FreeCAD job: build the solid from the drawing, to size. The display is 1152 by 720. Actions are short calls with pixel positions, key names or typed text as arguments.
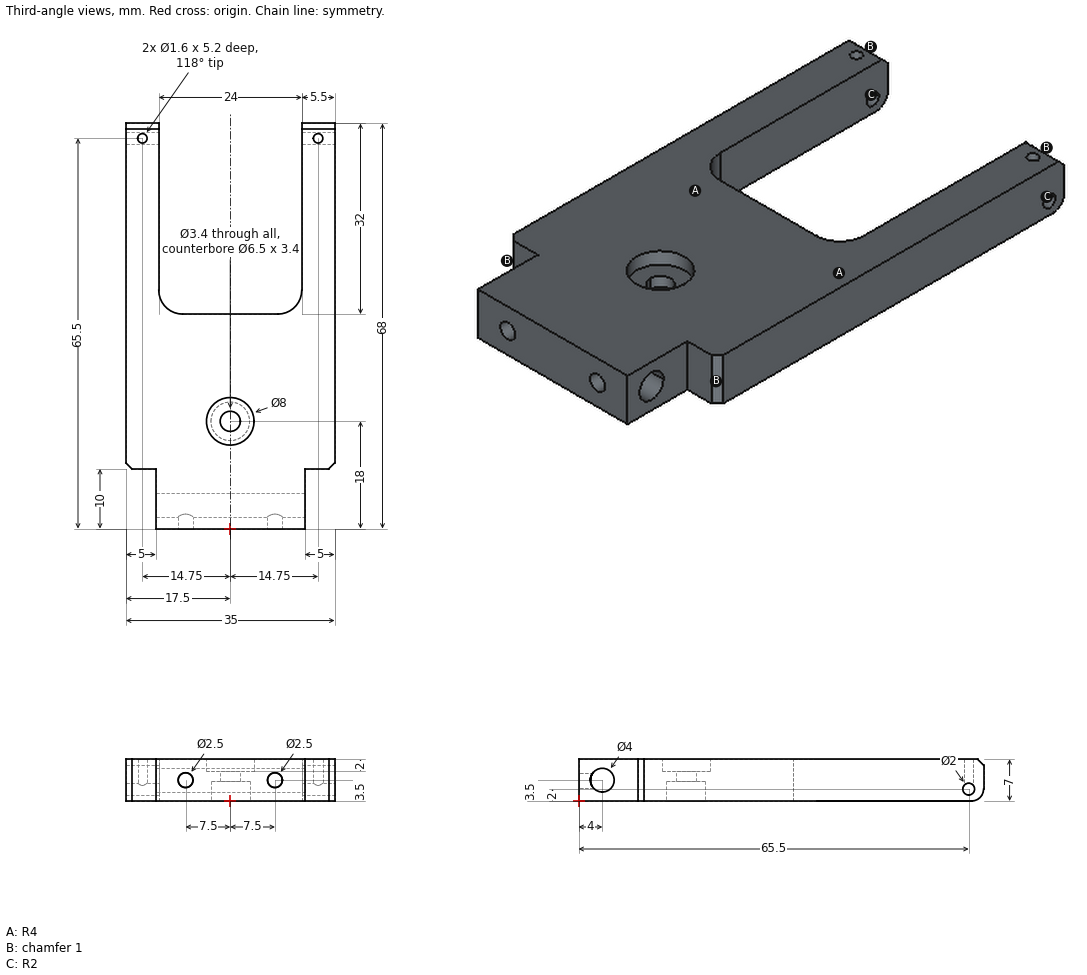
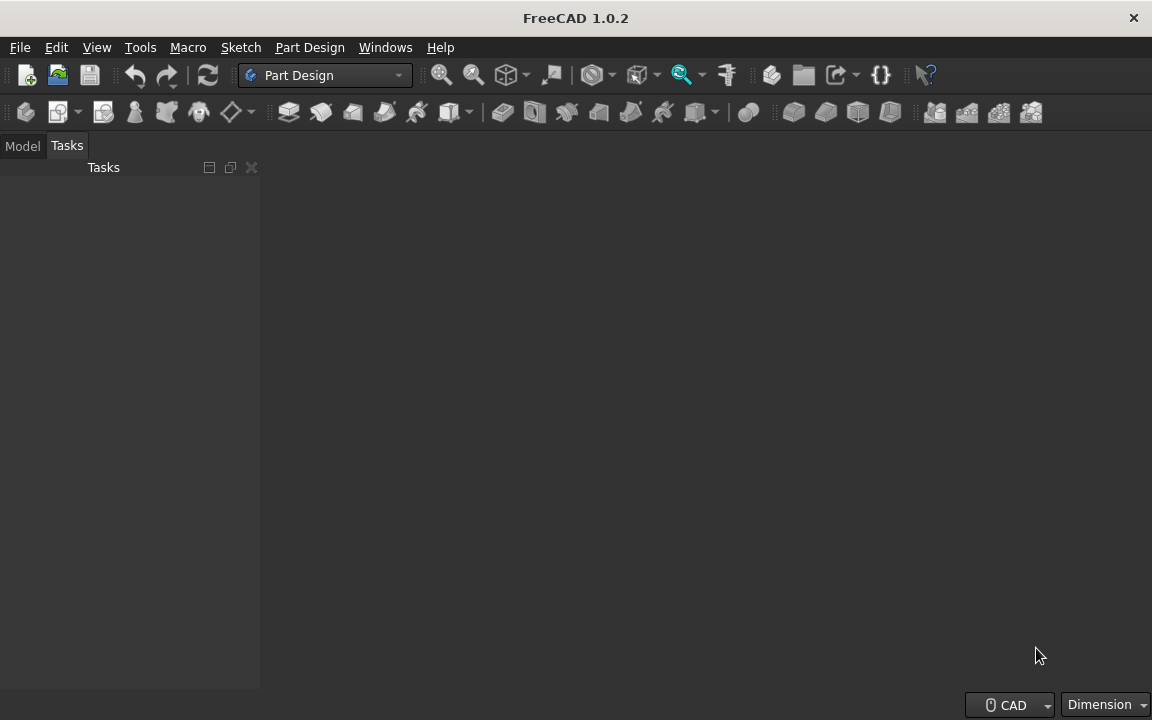
key(ctrl+n)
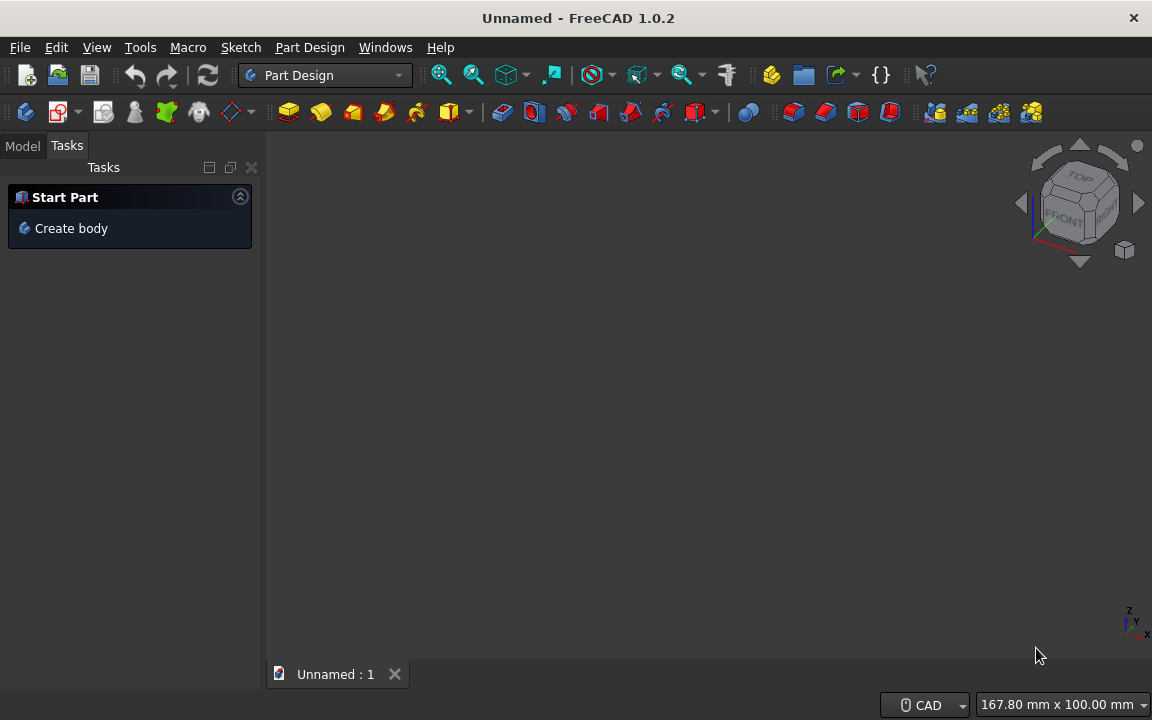
click(58, 112)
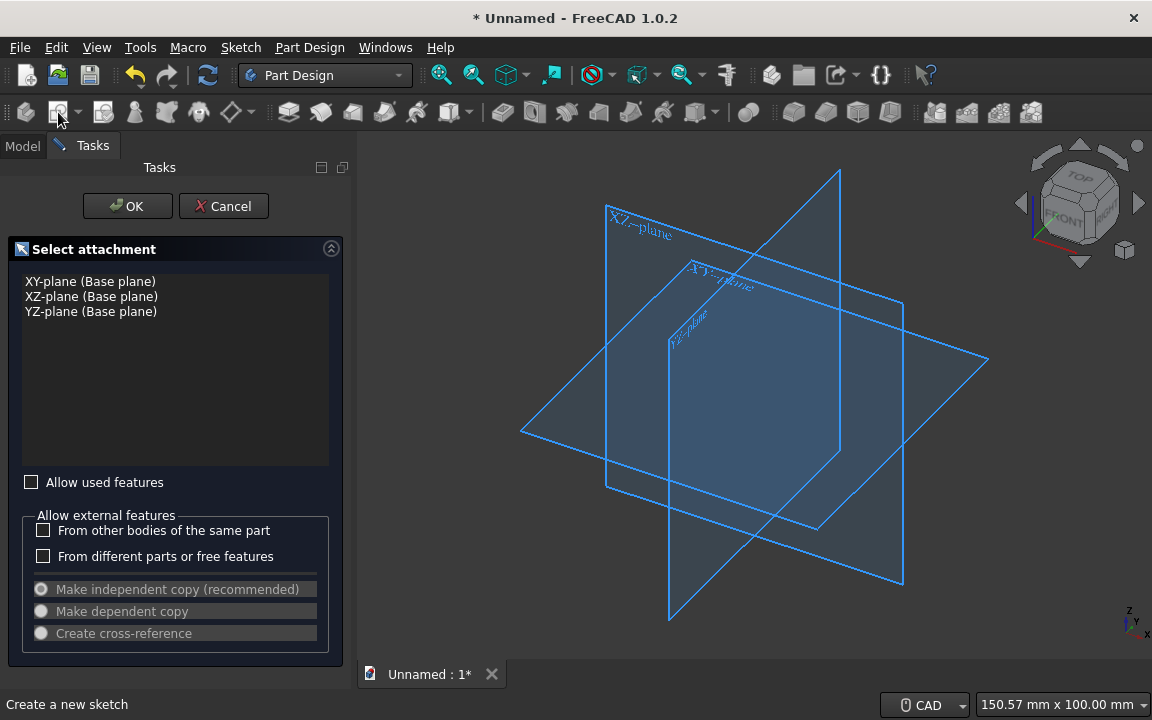
click(82, 282)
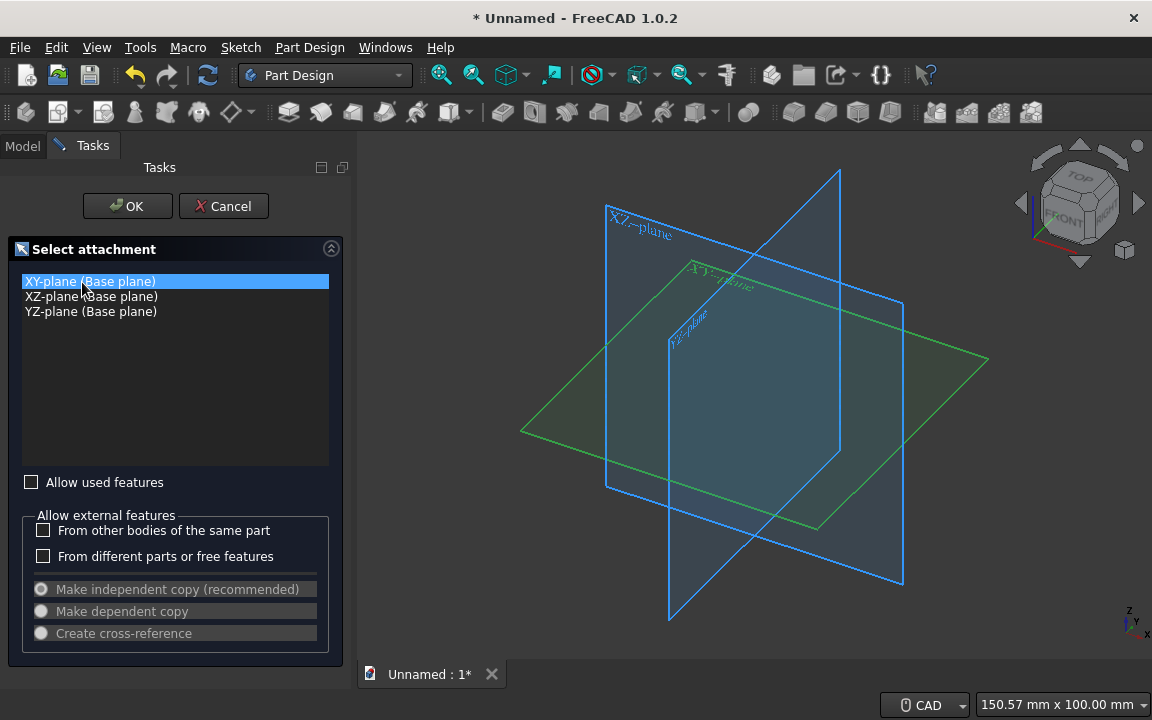
click(128, 206)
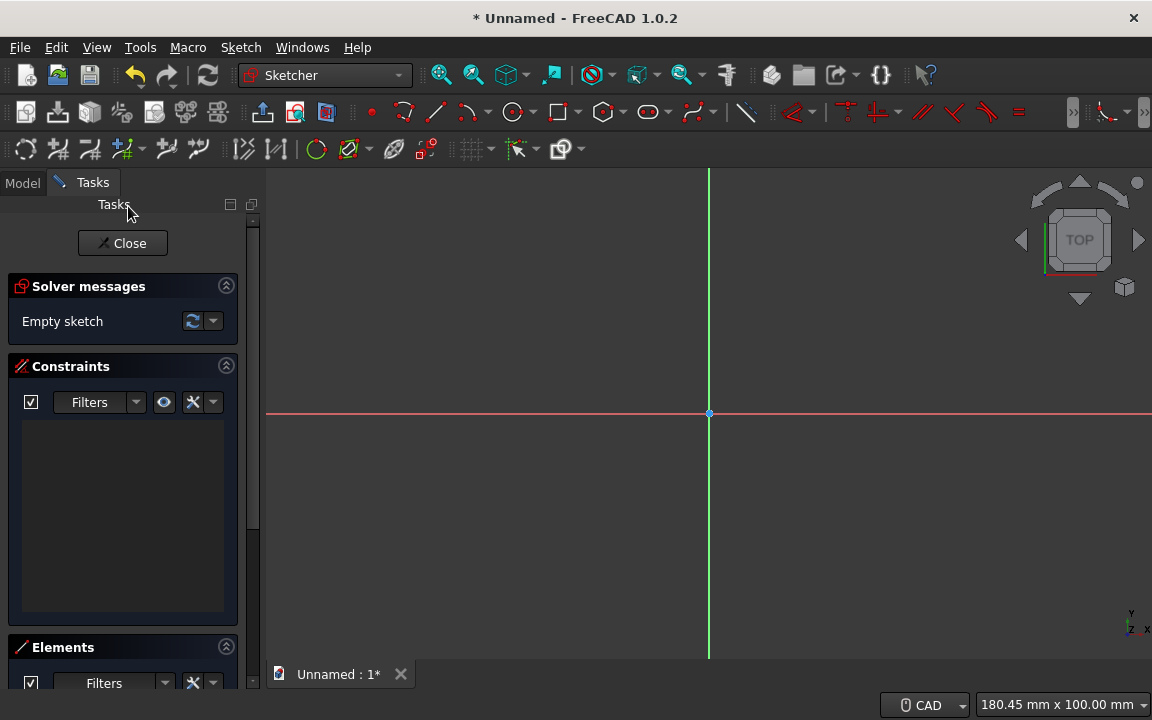
scroll(501, 631, down, 2)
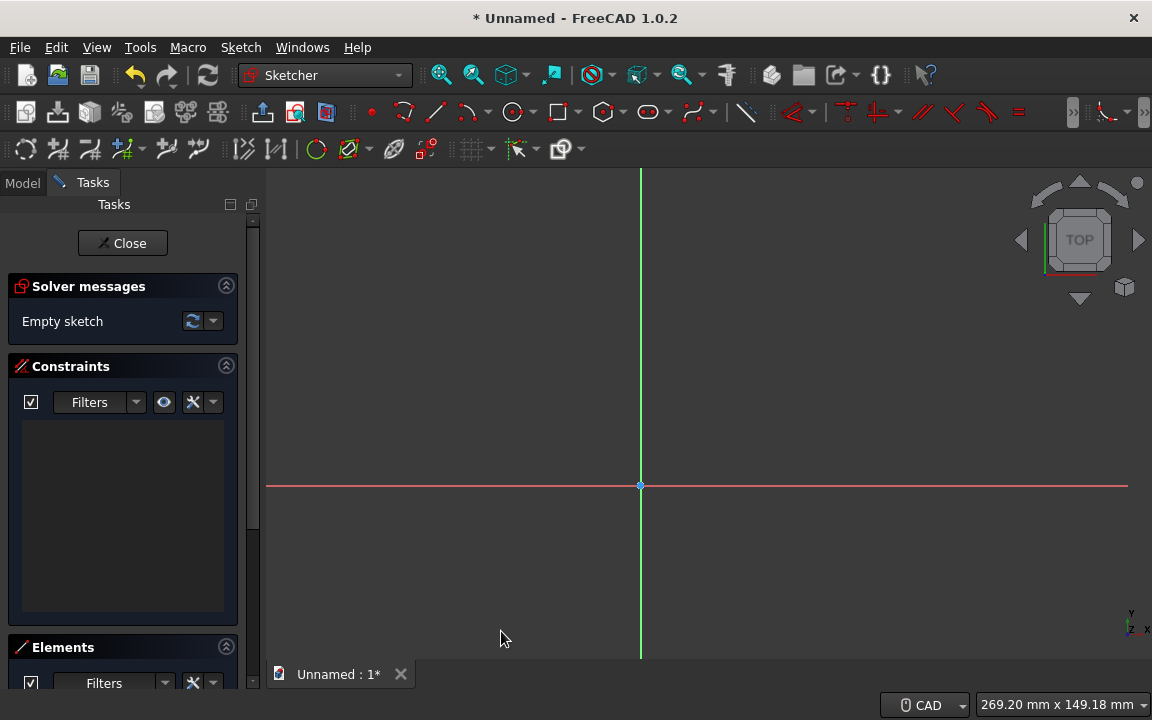
scroll(641, 293, up, 2)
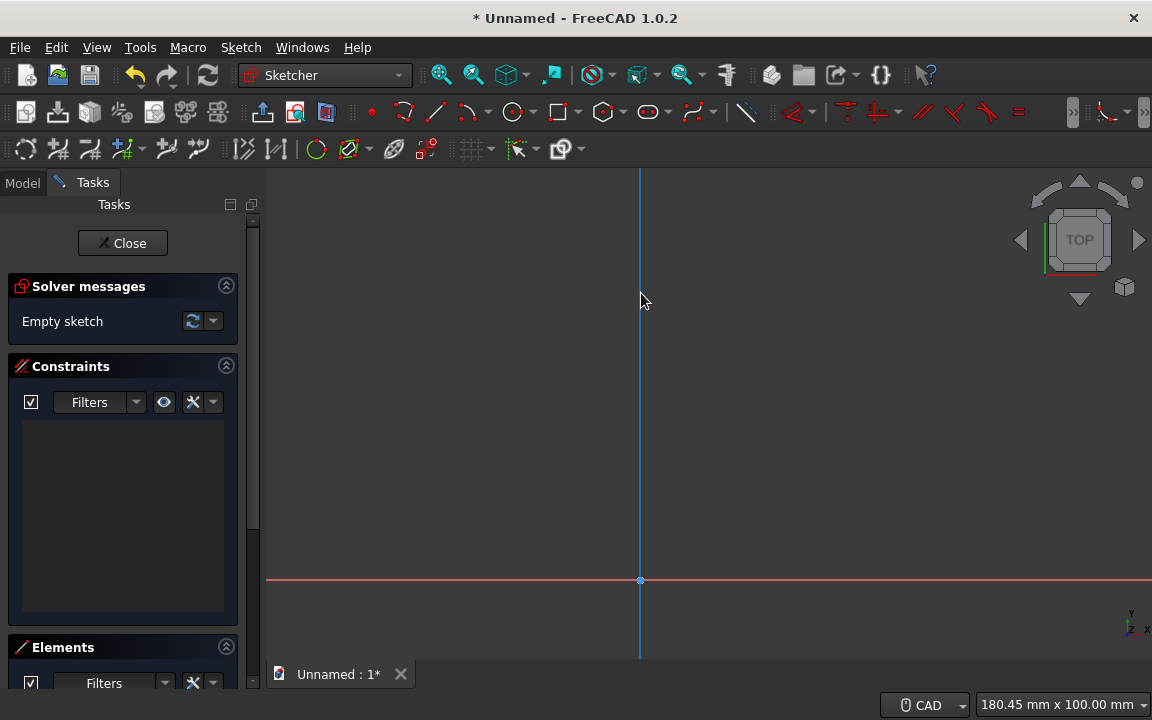
key(g)
key(m)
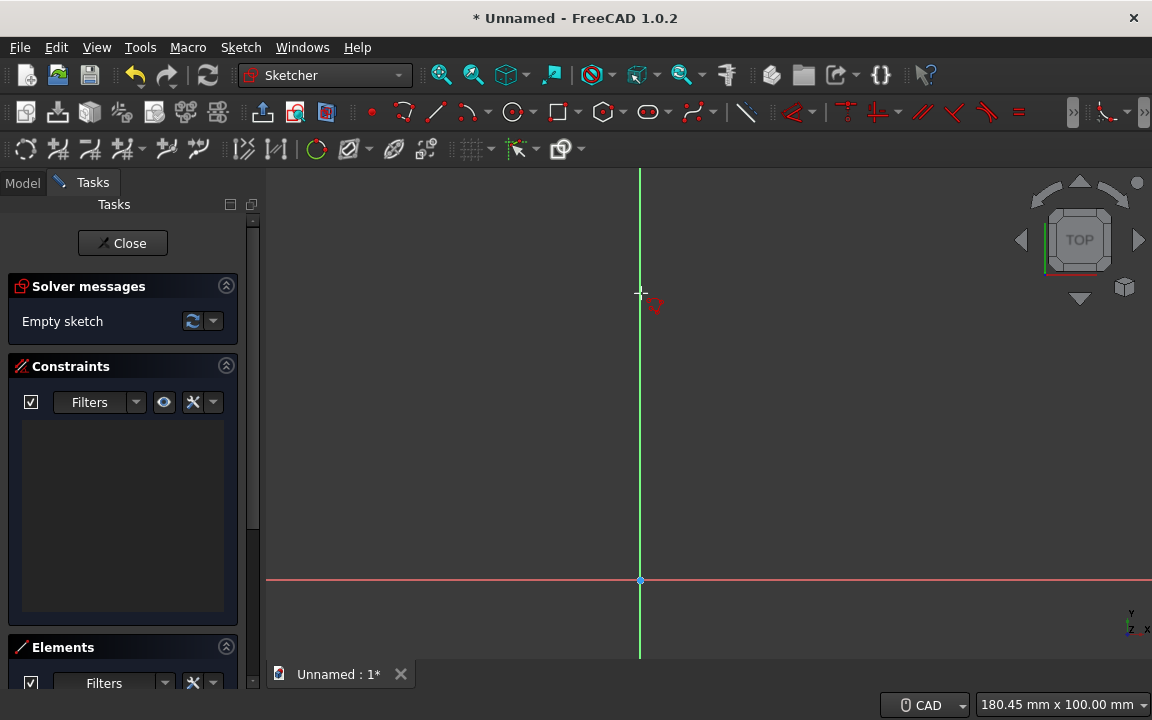
click(554, 580)
click(726, 571)
click(726, 246)
click(699, 246)
click(699, 403)
click(581, 403)
click(581, 246)
click(554, 246)
click(554, 580)
key(Escape)
key(Escape)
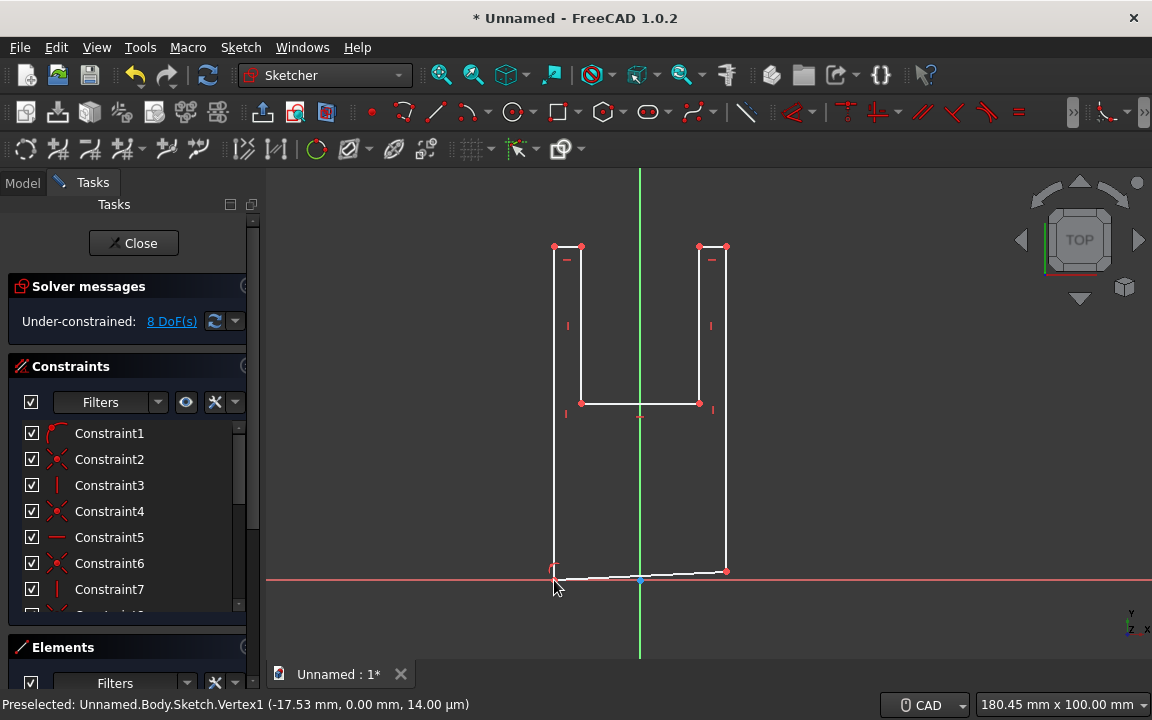
click(606, 578)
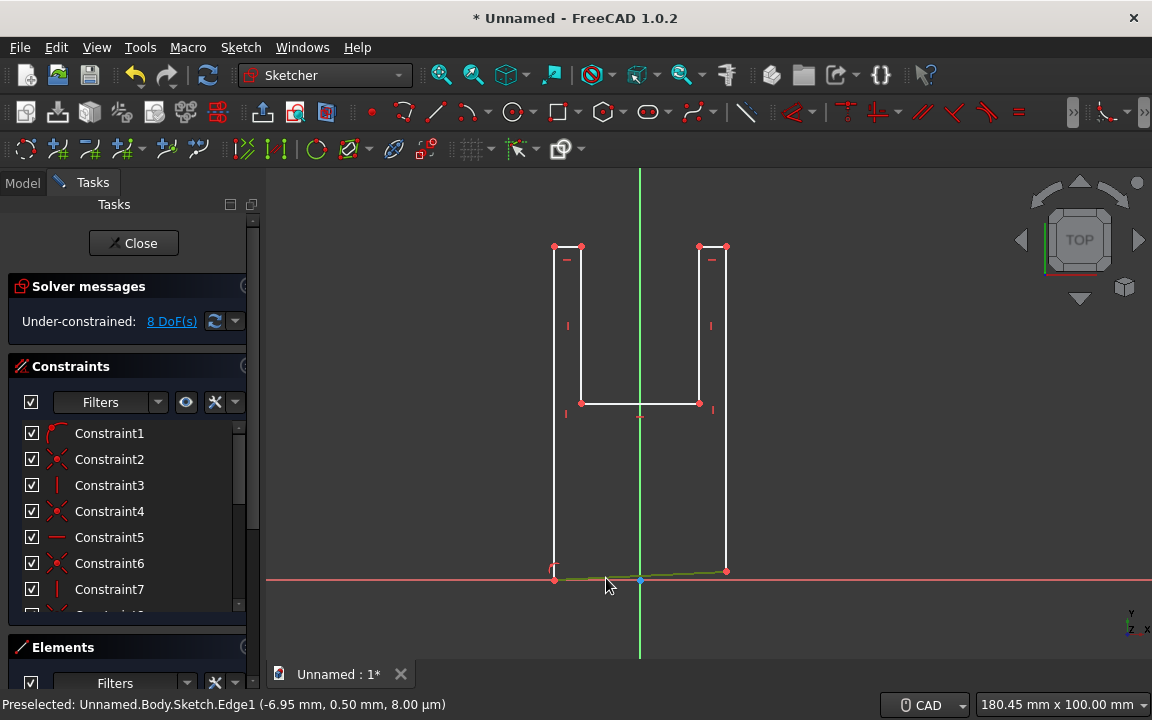
key(h)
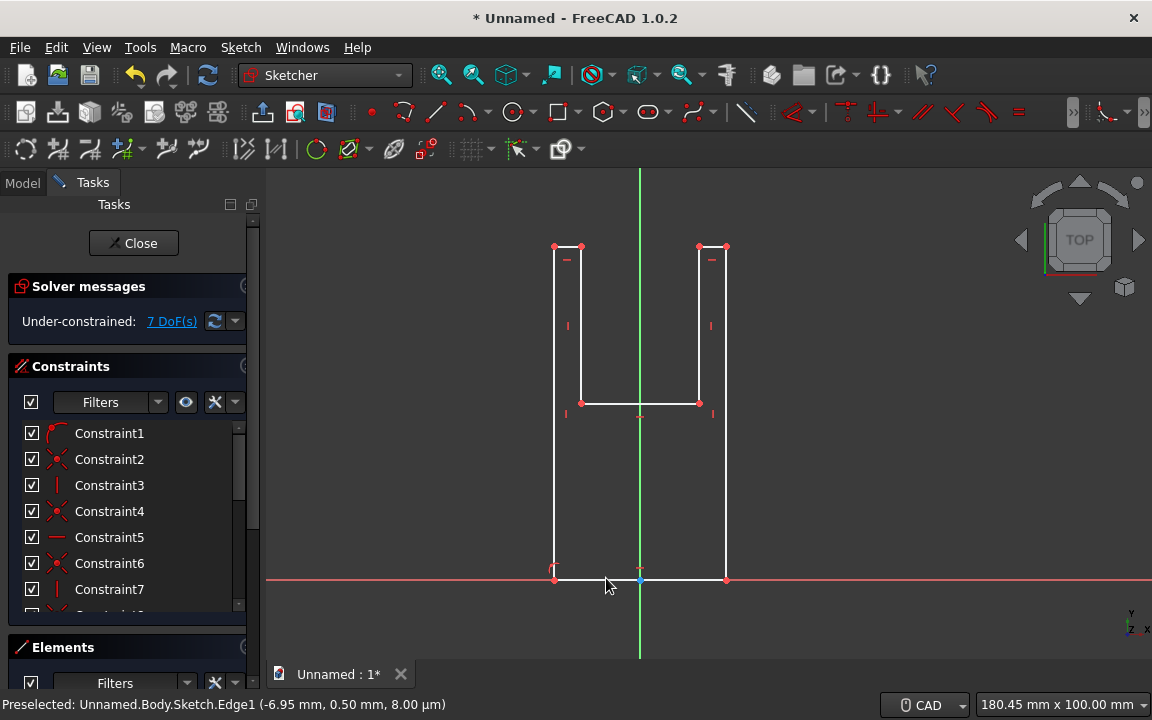
click(699, 247)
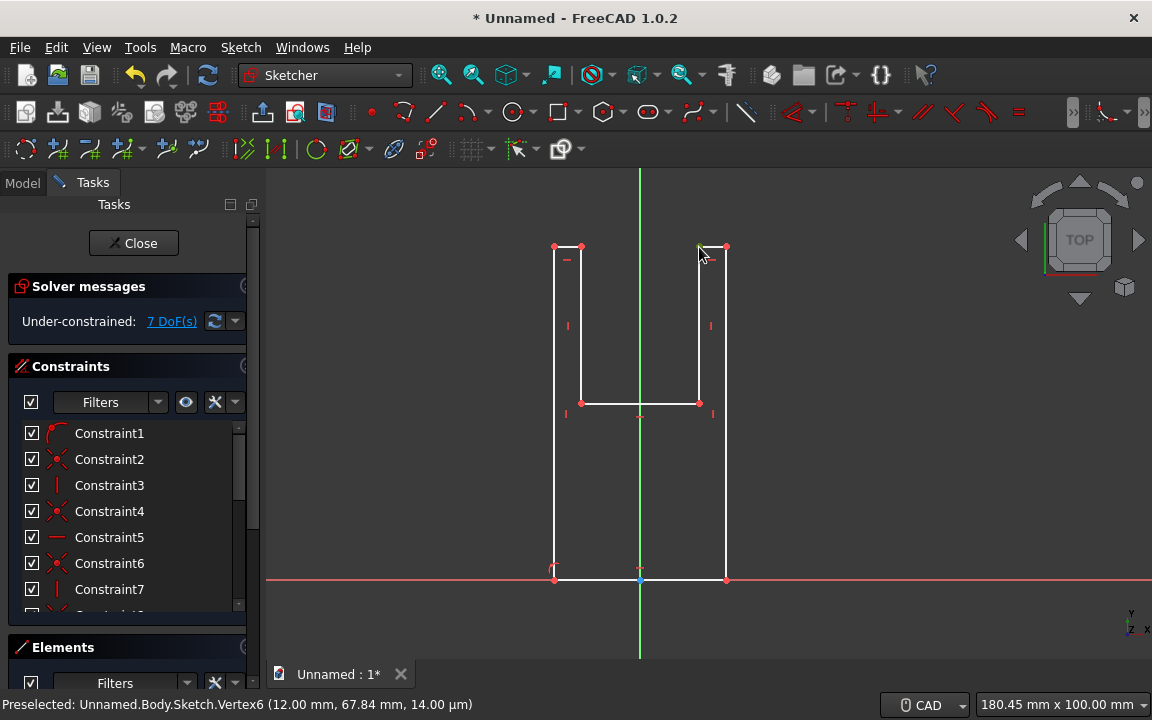
click(581, 247)